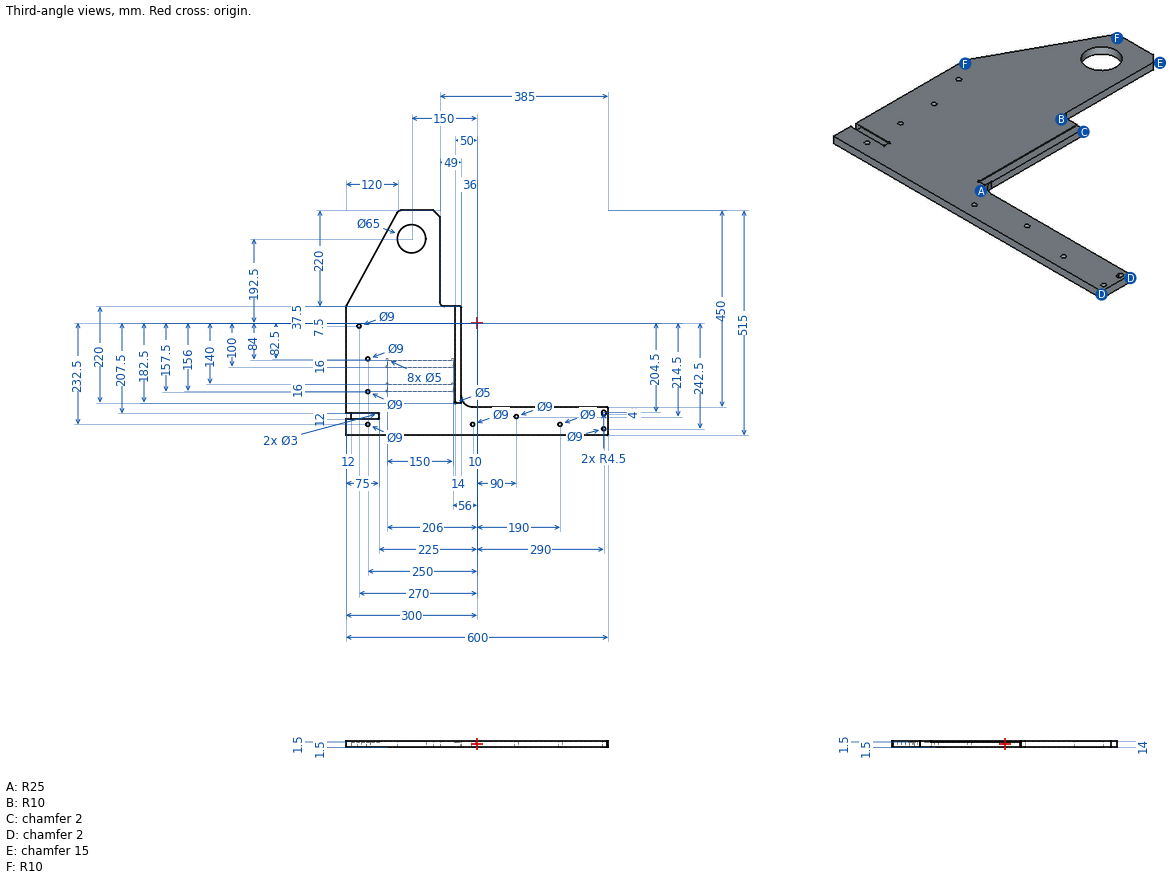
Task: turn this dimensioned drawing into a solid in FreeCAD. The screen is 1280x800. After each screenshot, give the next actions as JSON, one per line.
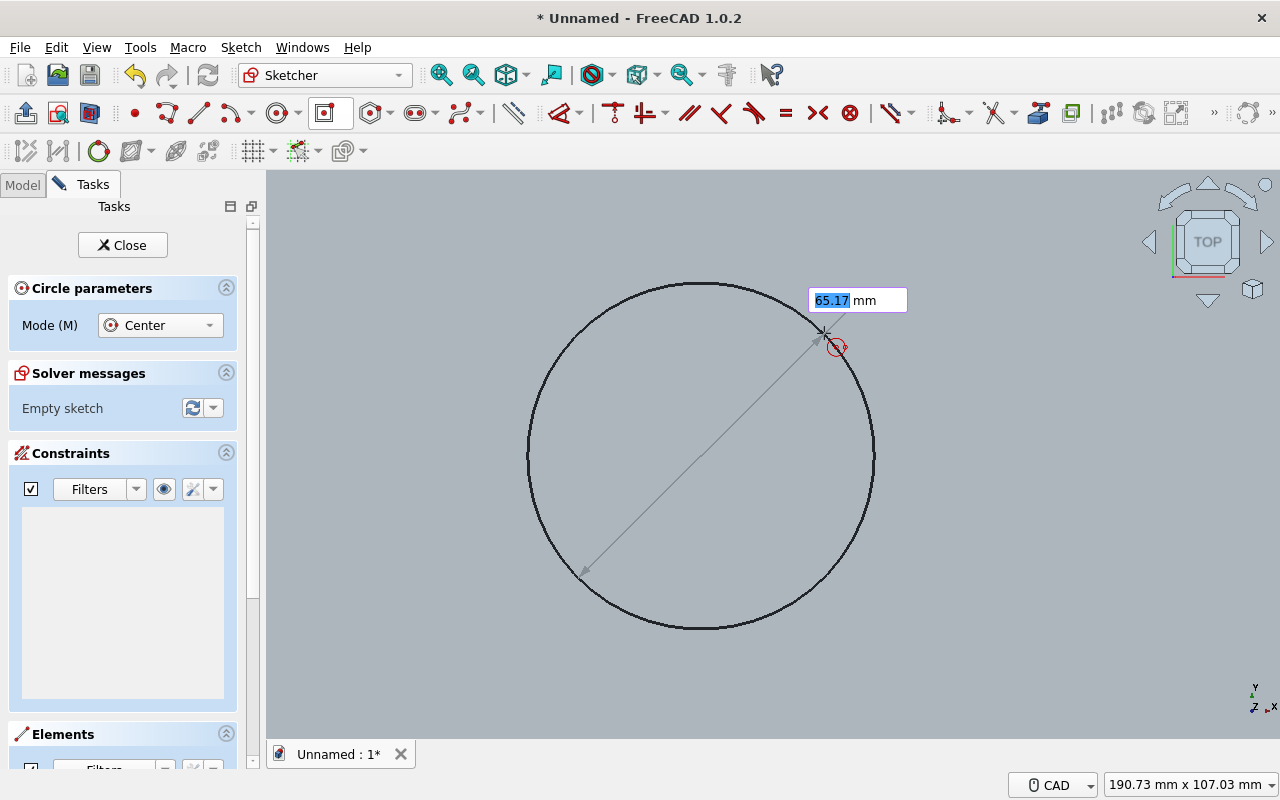
{"action": "type", "text": "65"}
{"action": "key", "text": "Return"}
{"action": "key", "text": "Escape"}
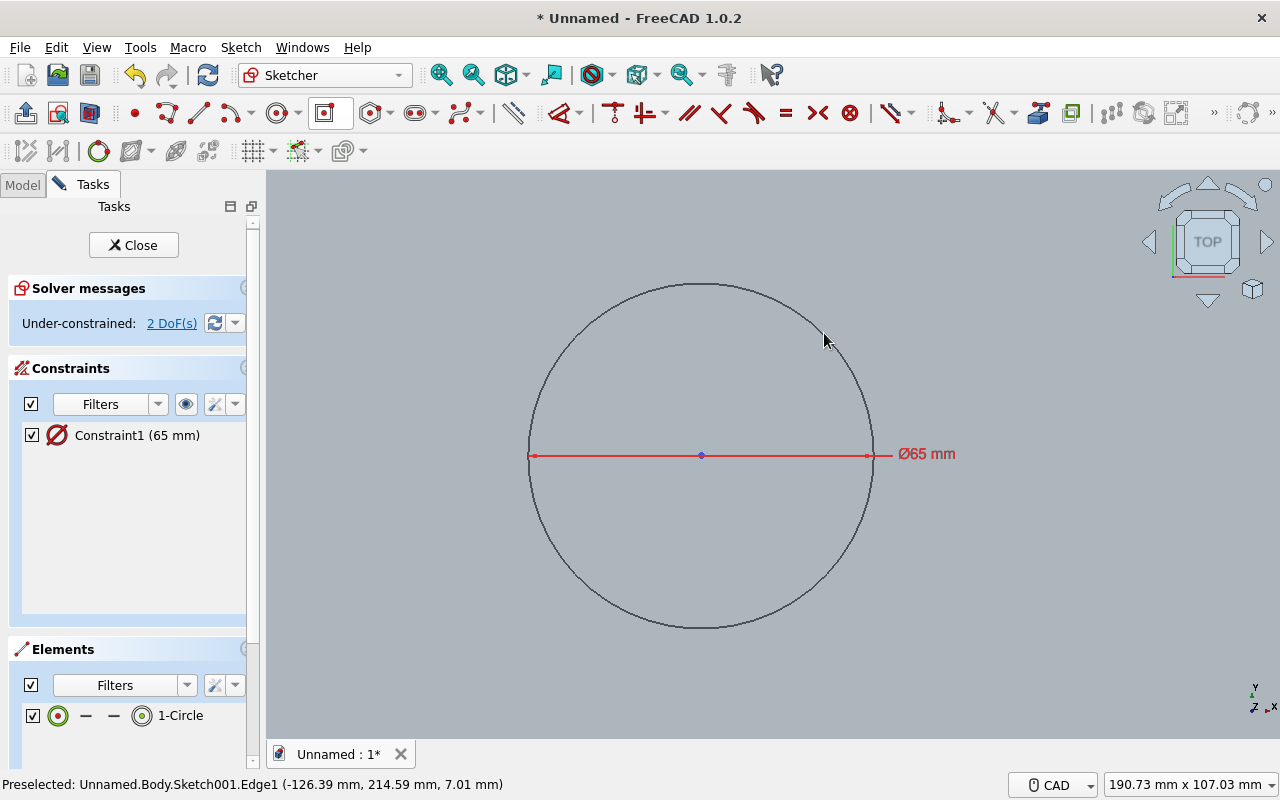
{"action": "left_click", "coordinate": [701, 456]}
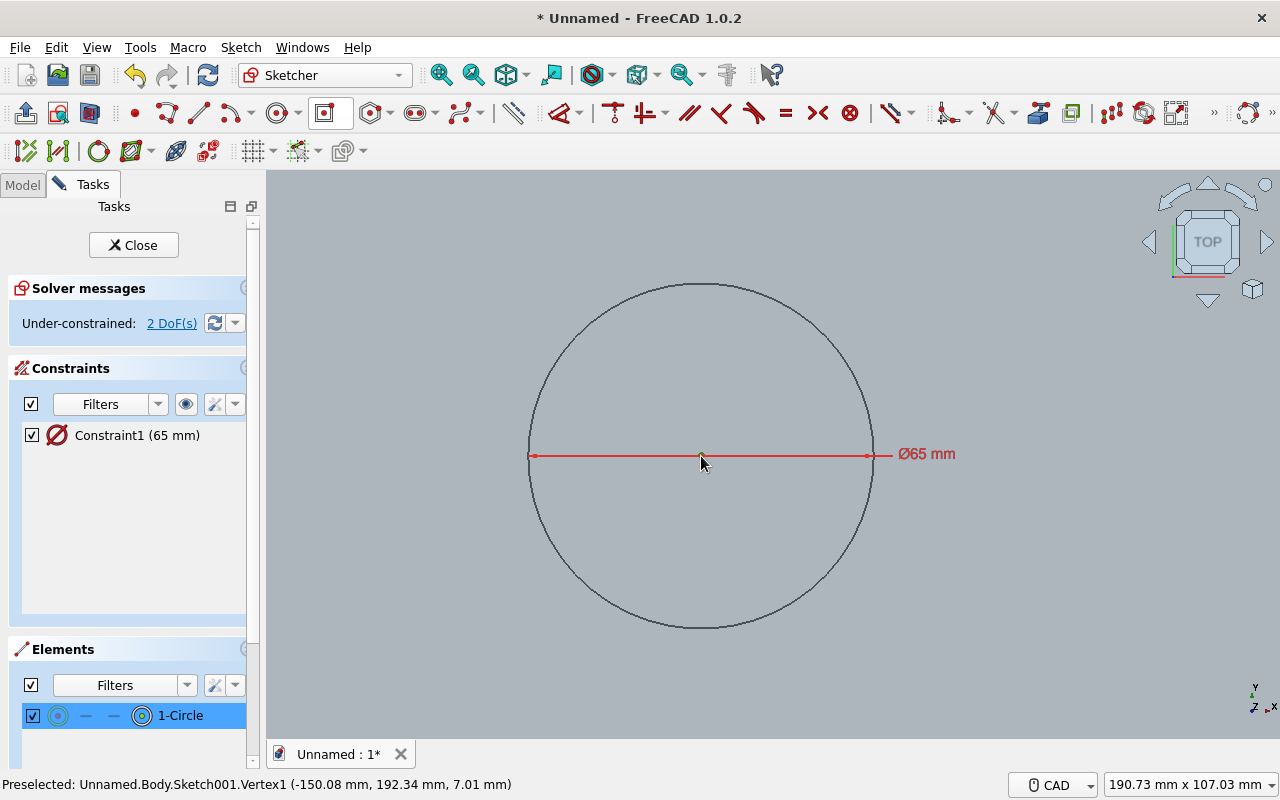
{"action": "key", "text": "l"}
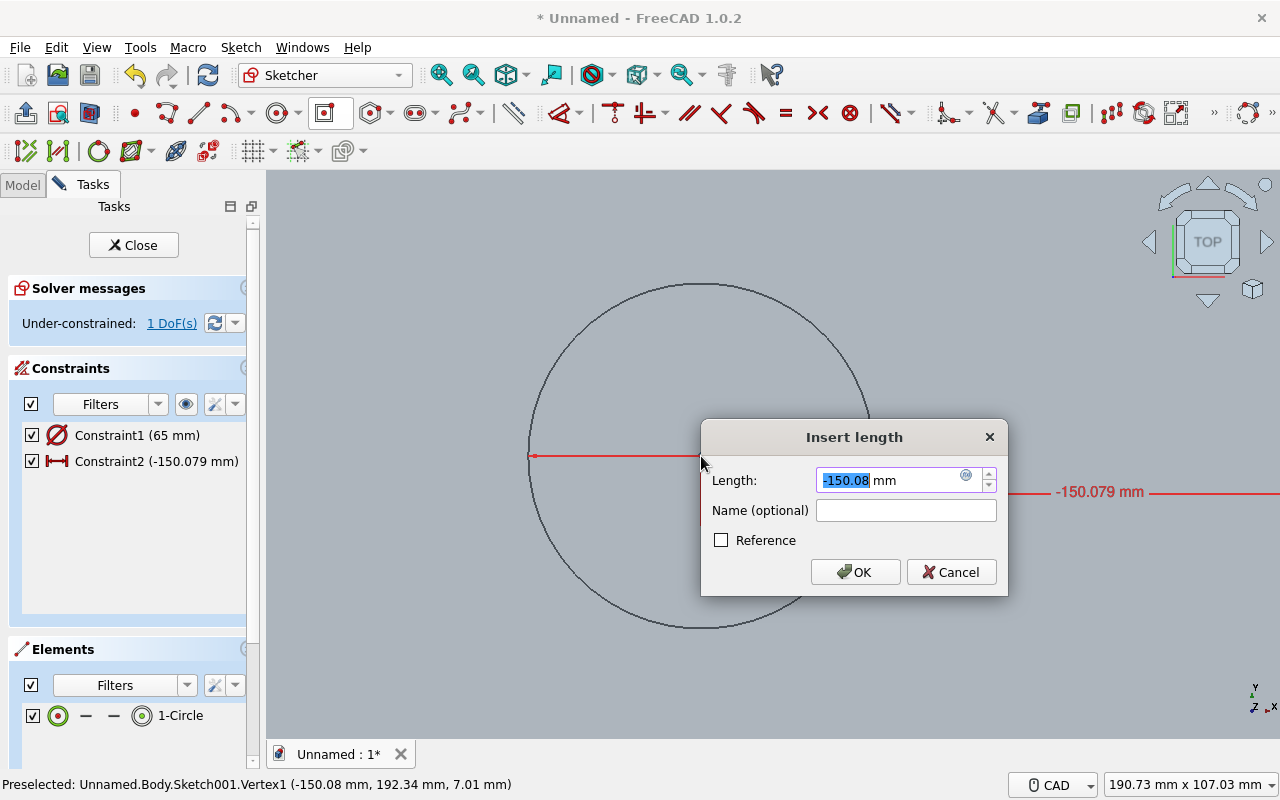
{"action": "type", "text": "-150"}
{"action": "key", "text": "Return"}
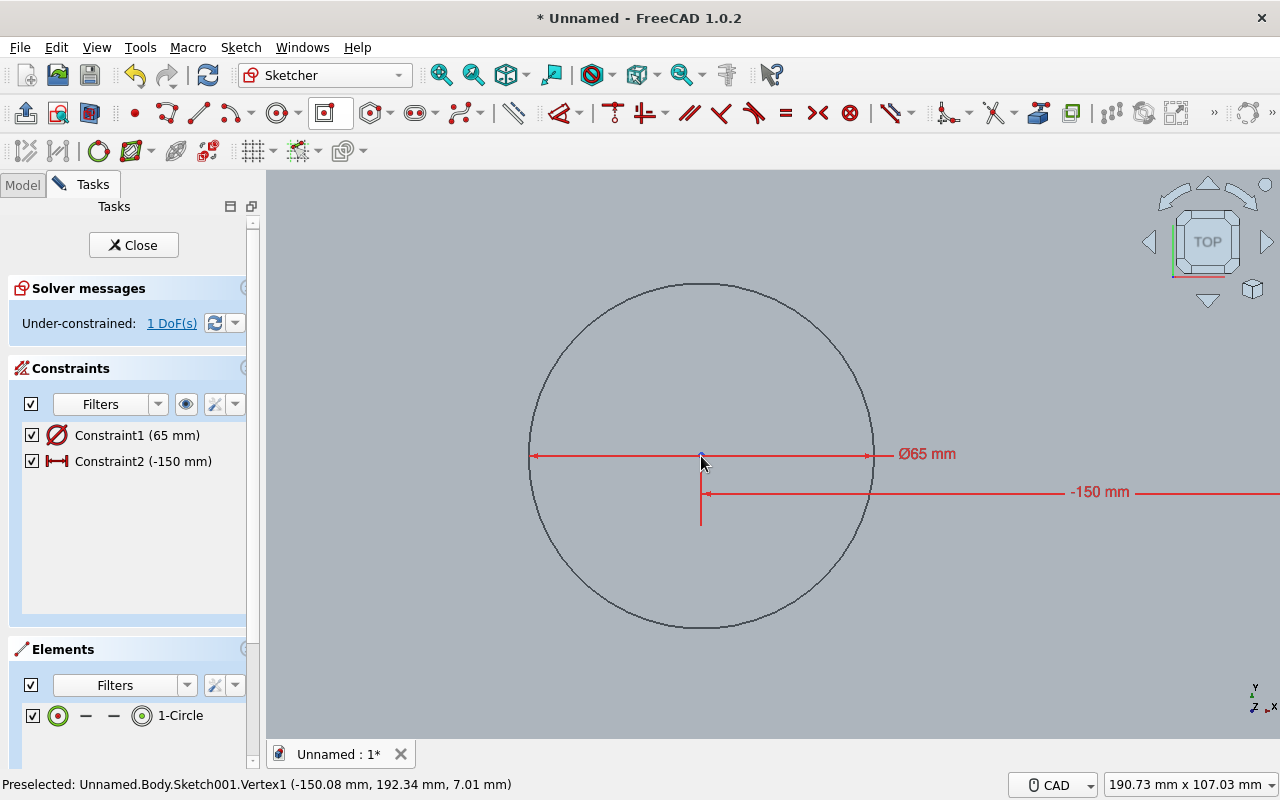
{"action": "left_click", "coordinate": [701, 456]}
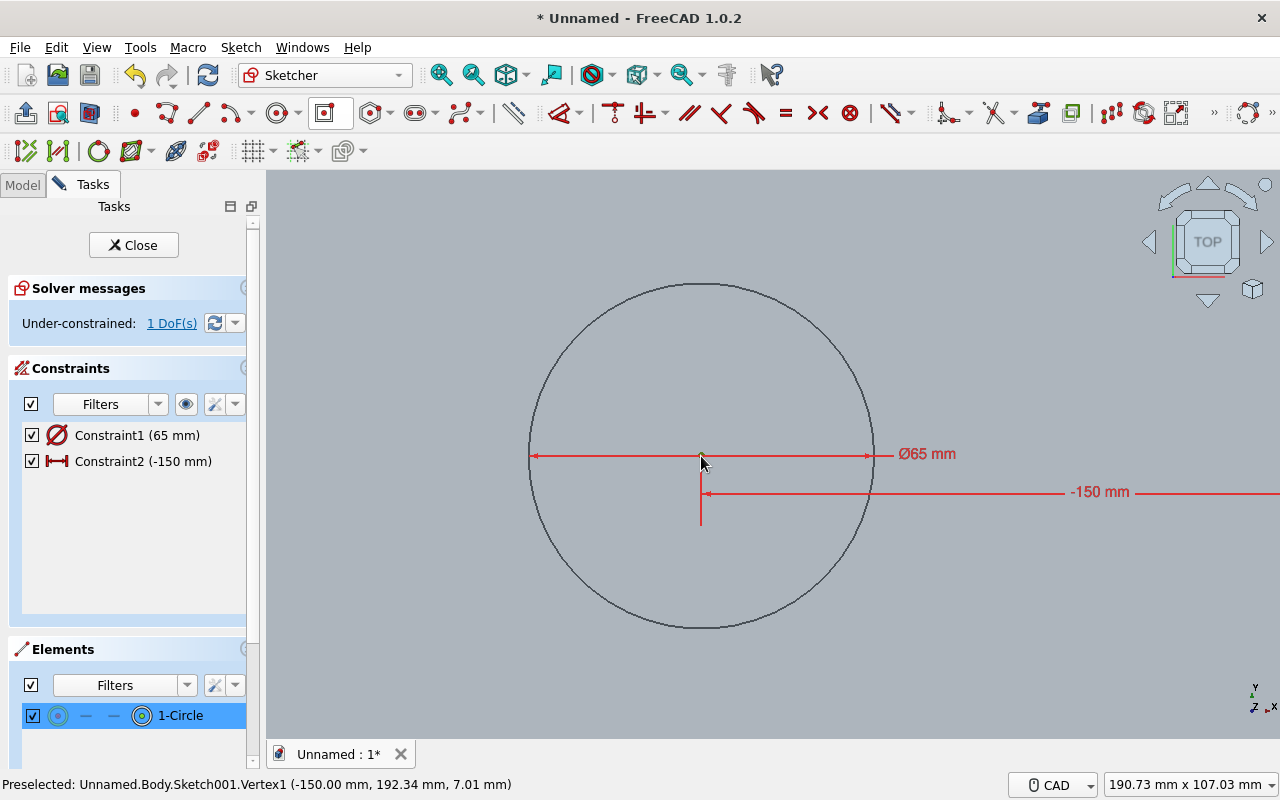
{"action": "left_click", "coordinate": [582, 114]}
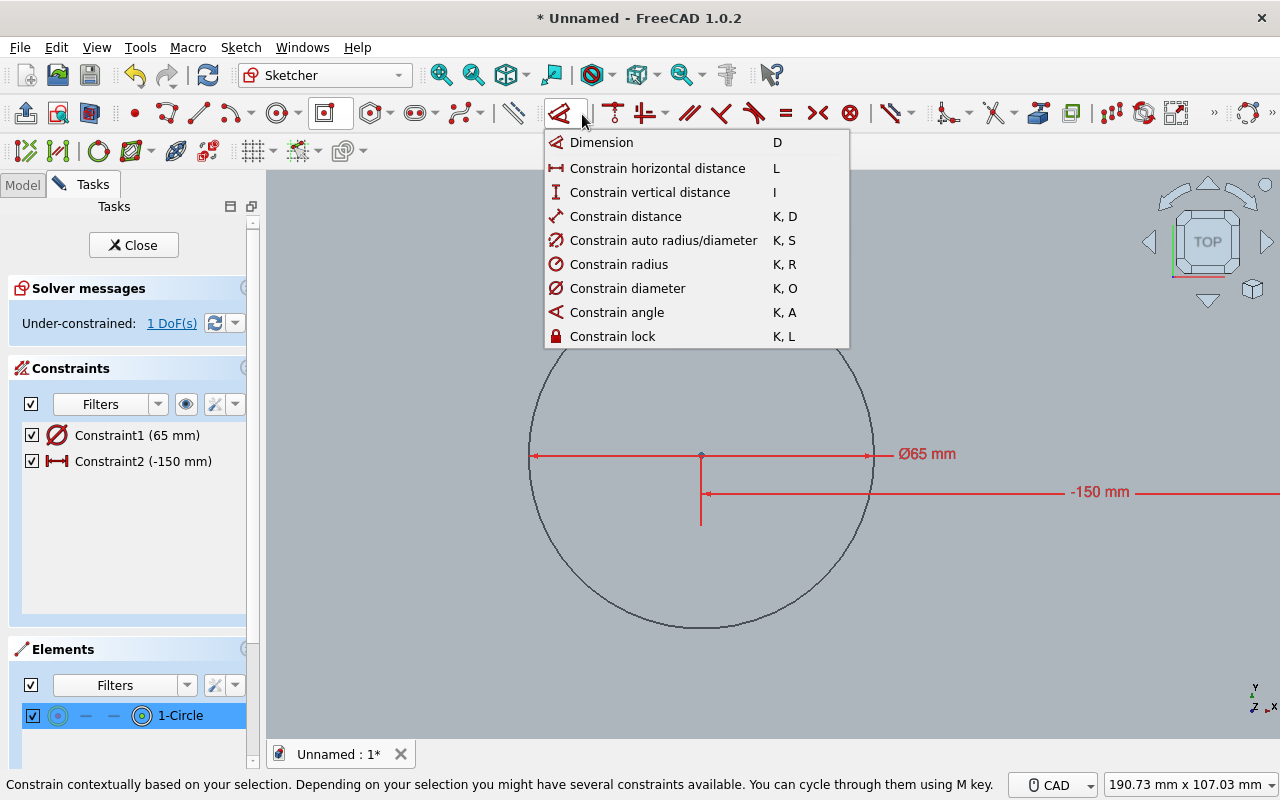
{"action": "left_click", "coordinate": [697, 192]}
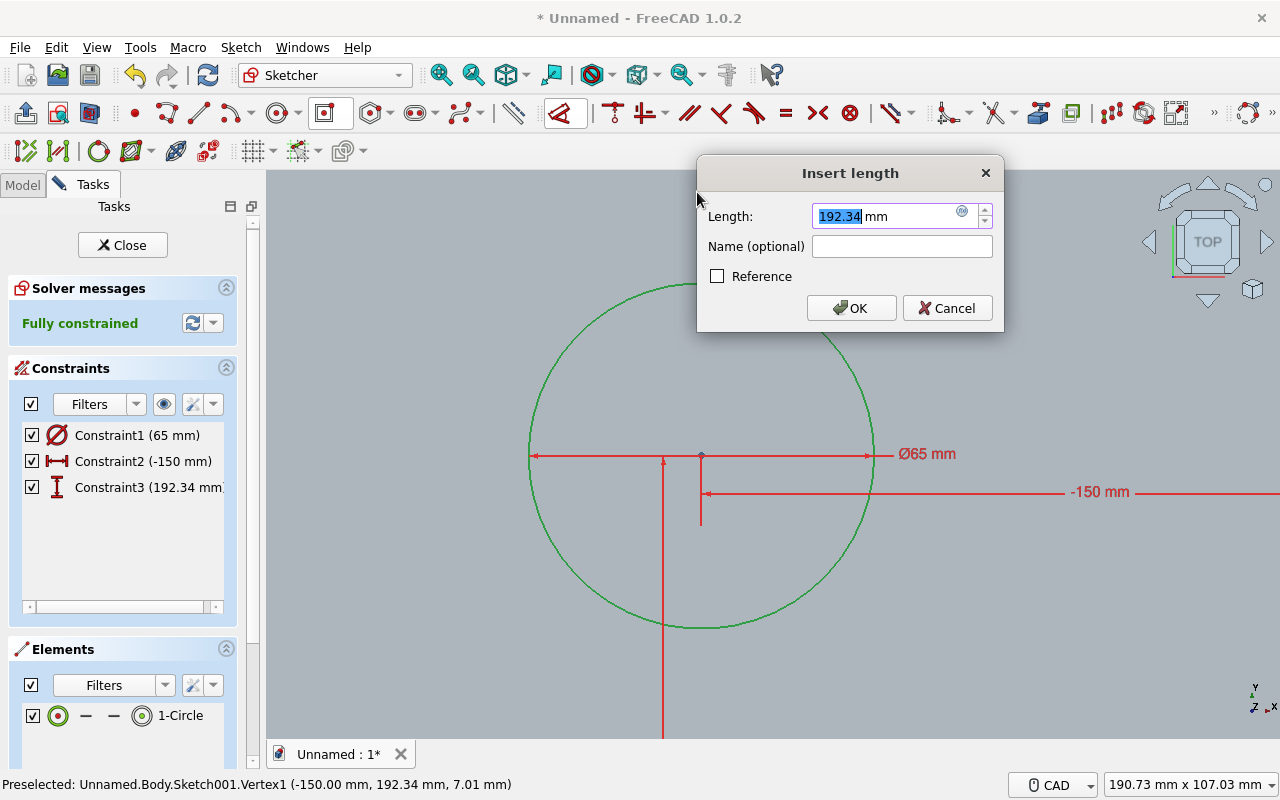
{"action": "type", "text": "192.5"}
{"action": "key", "text": "Return"}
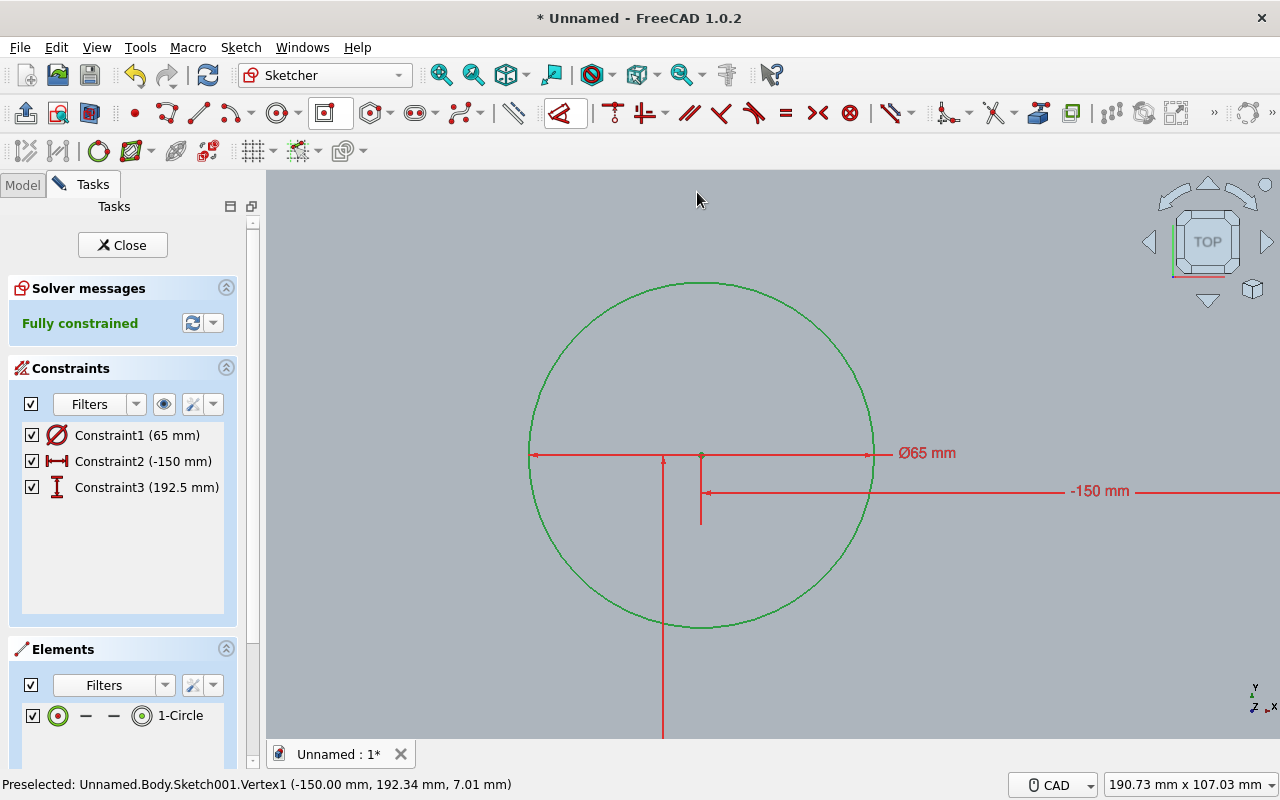
{"action": "left_click", "coordinate": [123, 245]}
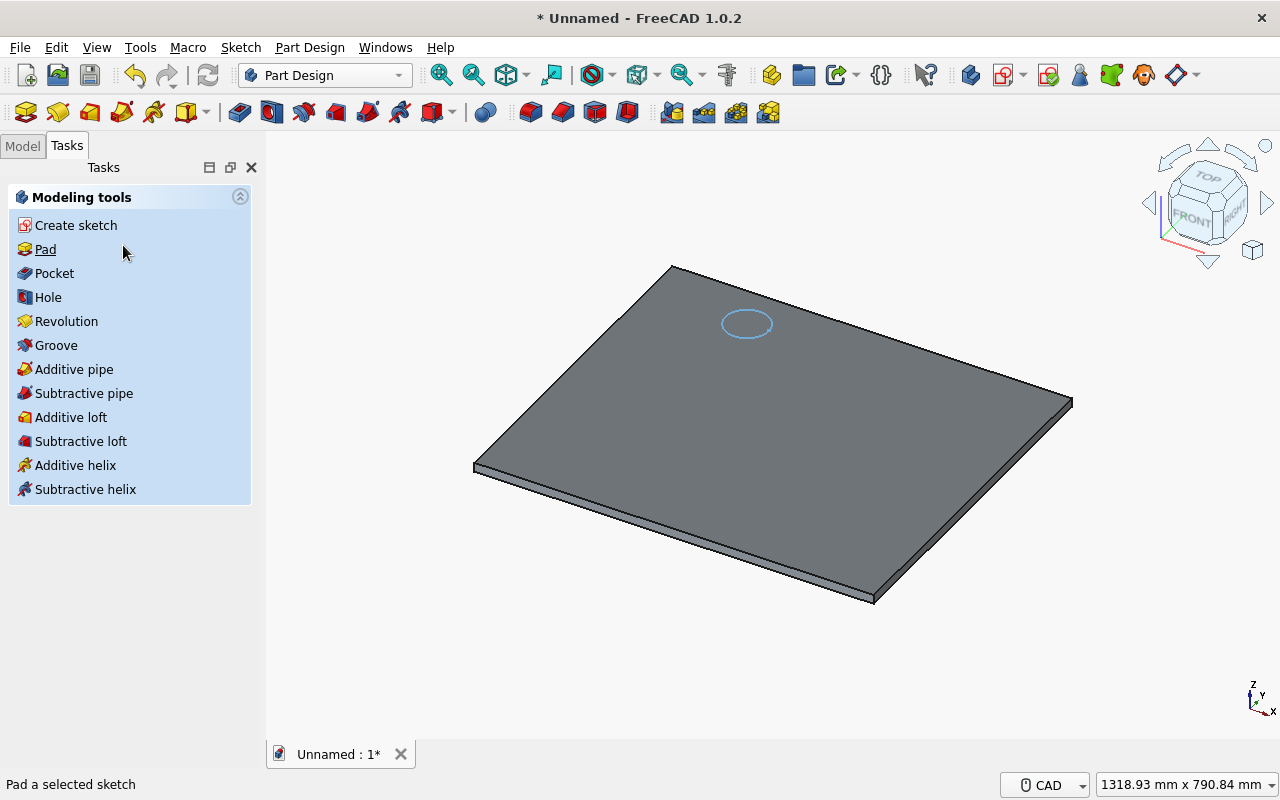
{"action": "left_click", "coordinate": [240, 112]}